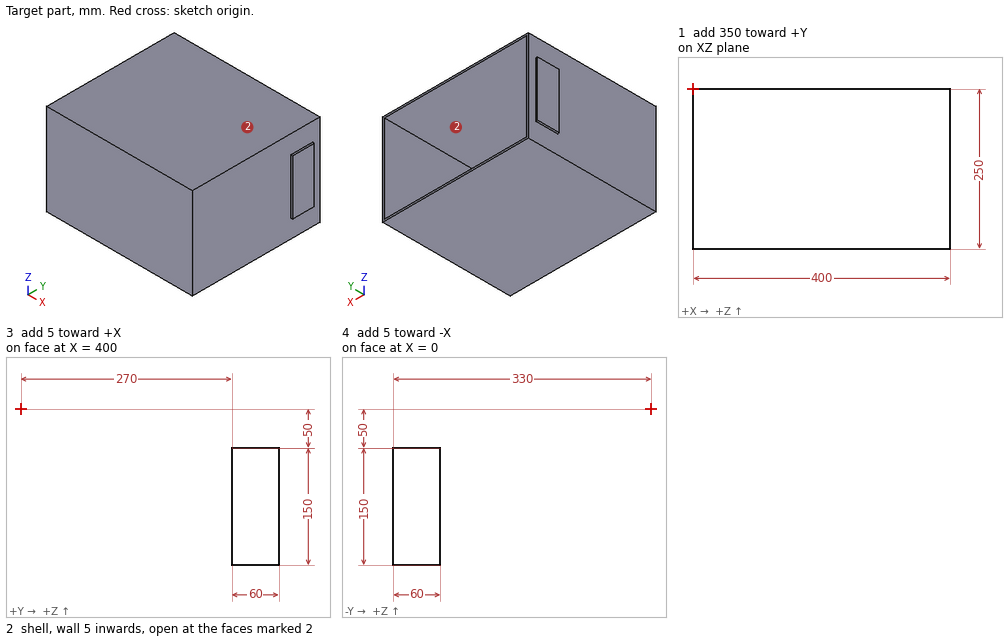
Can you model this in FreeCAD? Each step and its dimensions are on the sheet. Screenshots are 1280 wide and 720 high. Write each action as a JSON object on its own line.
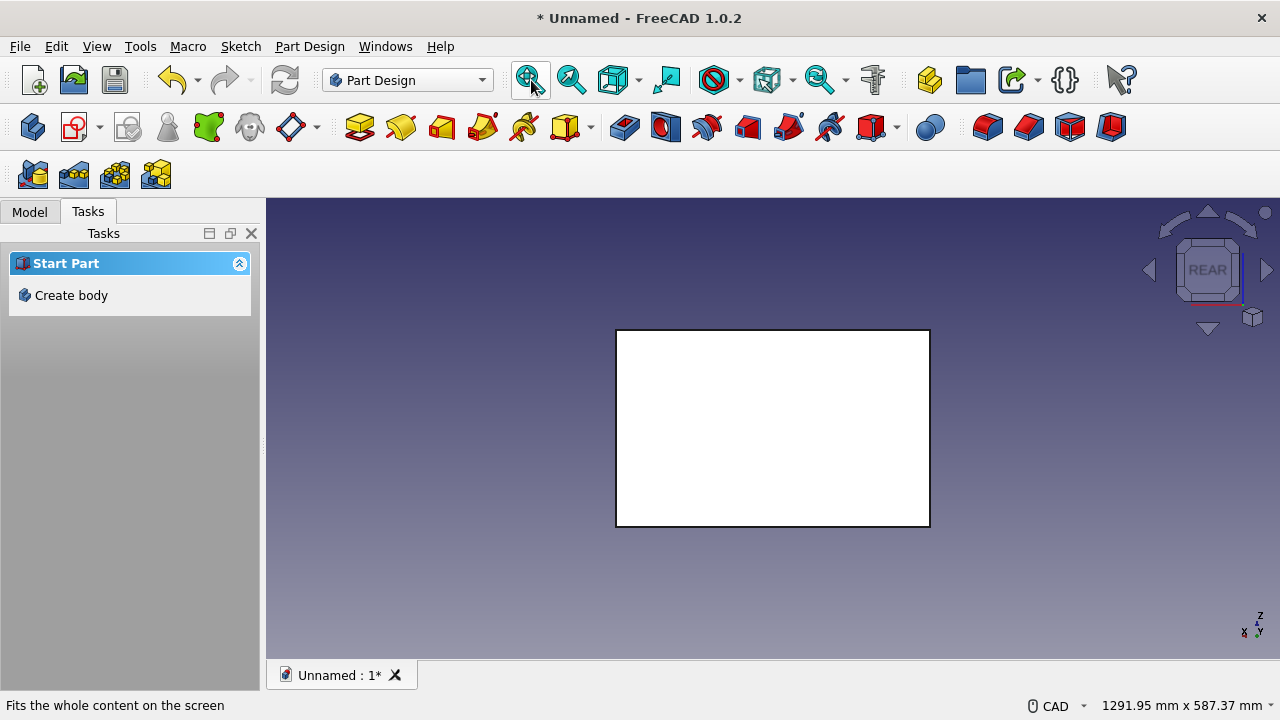
{"action": "key", "text": "v f"}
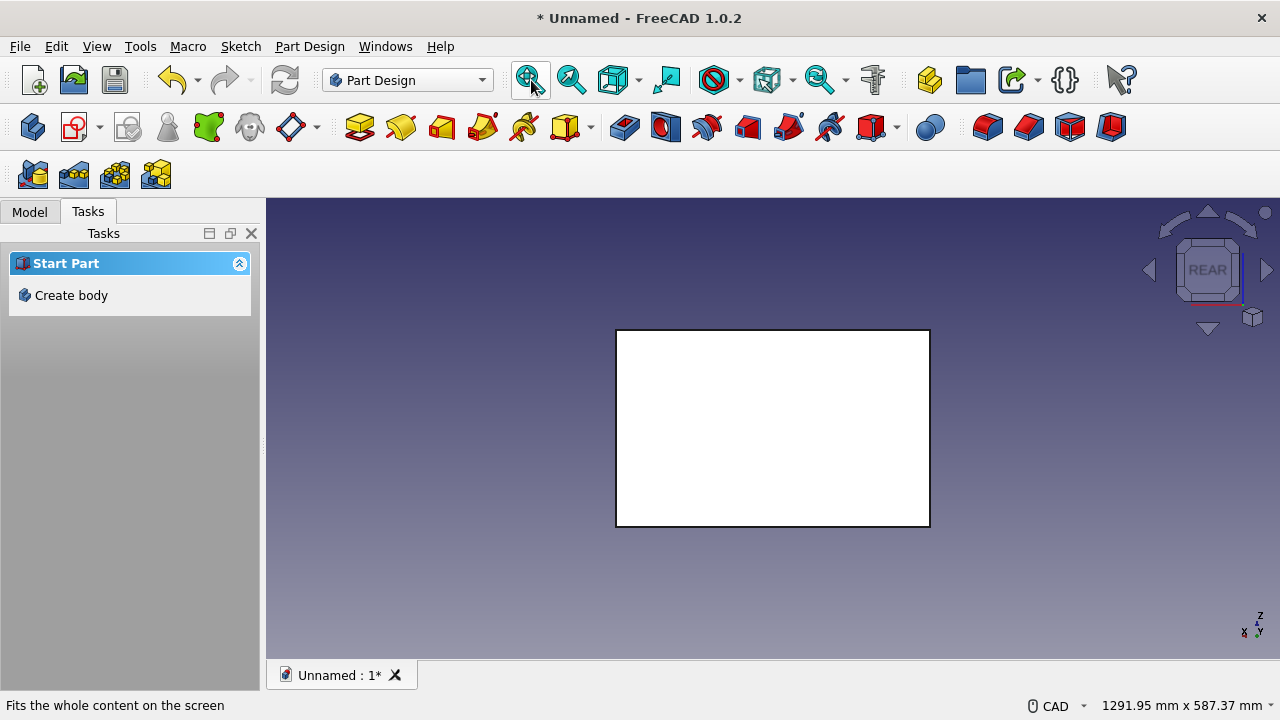
{"action": "left_click", "coordinate": [728, 428]}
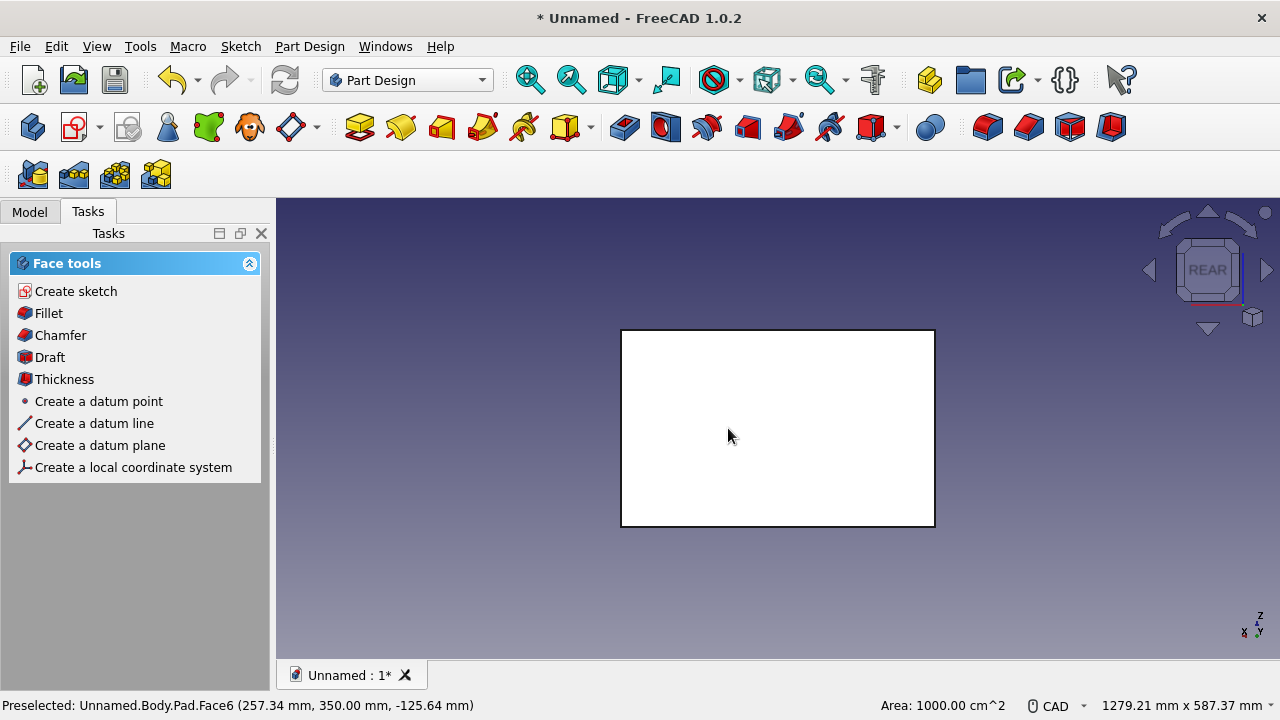
{"action": "left_click", "coordinate": [1111, 128]}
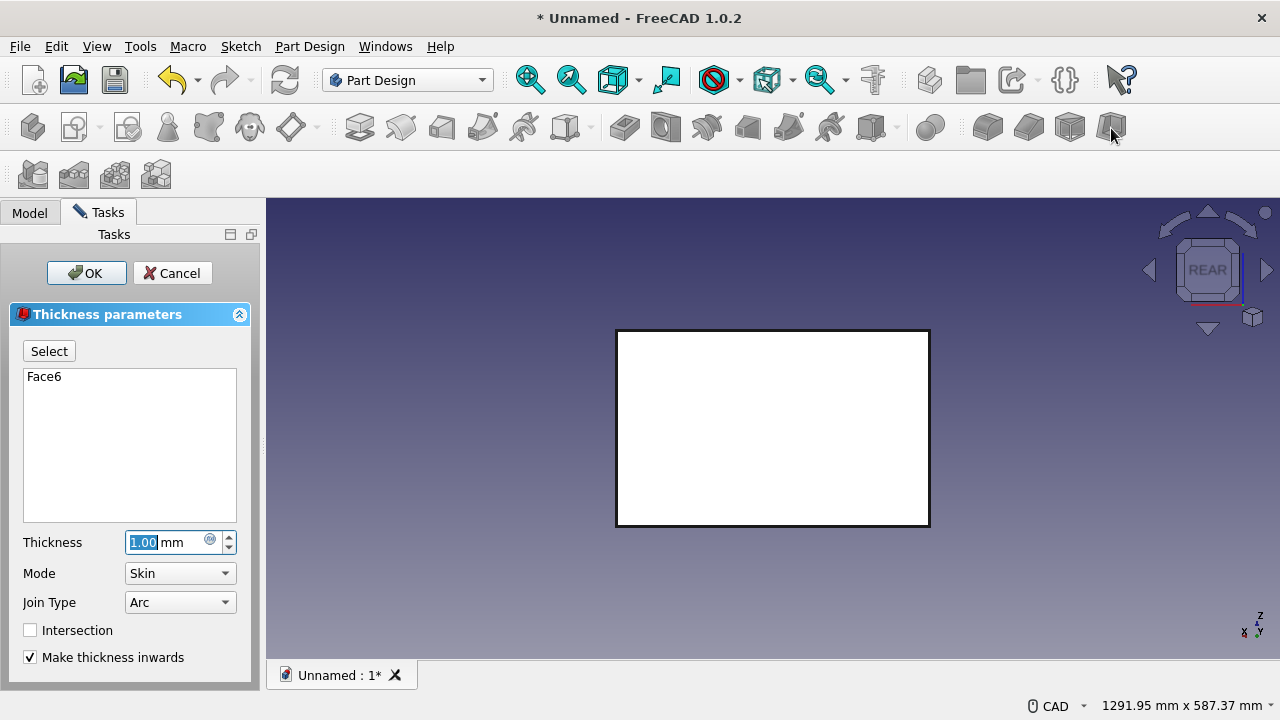
{"action": "type", "text": "5"}
{"action": "key", "text": "Tab"}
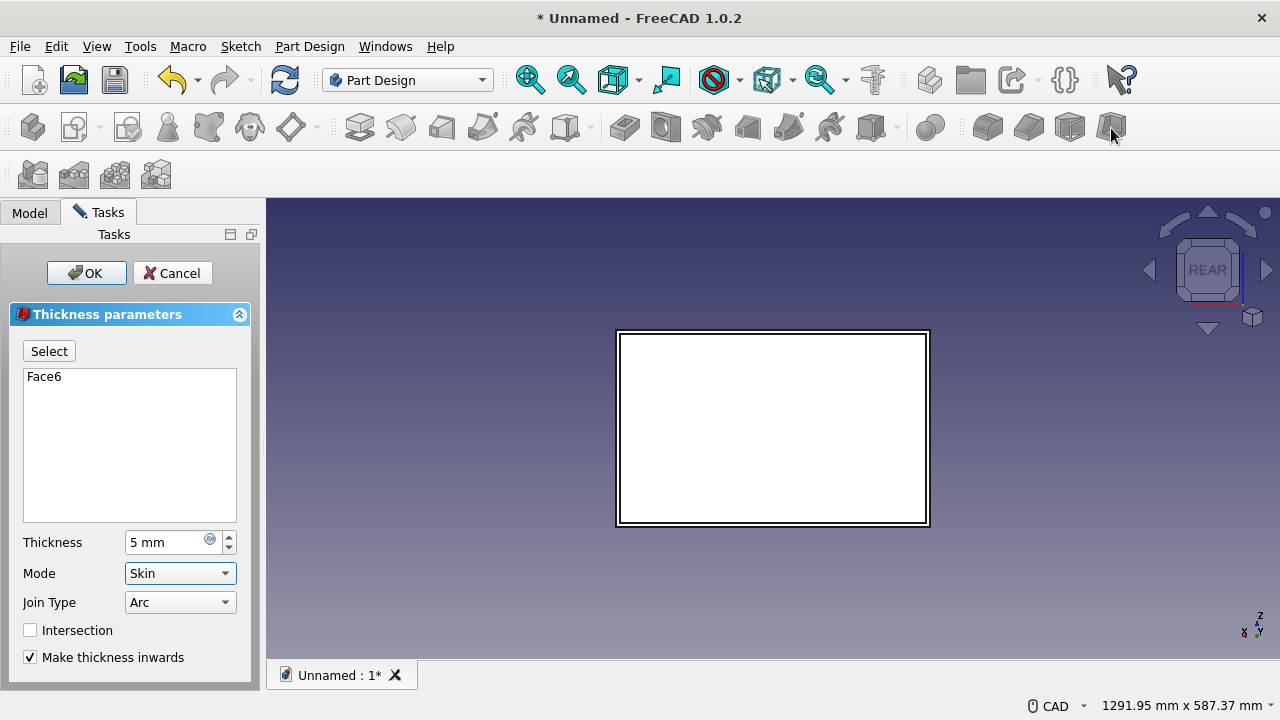
{"action": "left_click", "coordinate": [181, 602]}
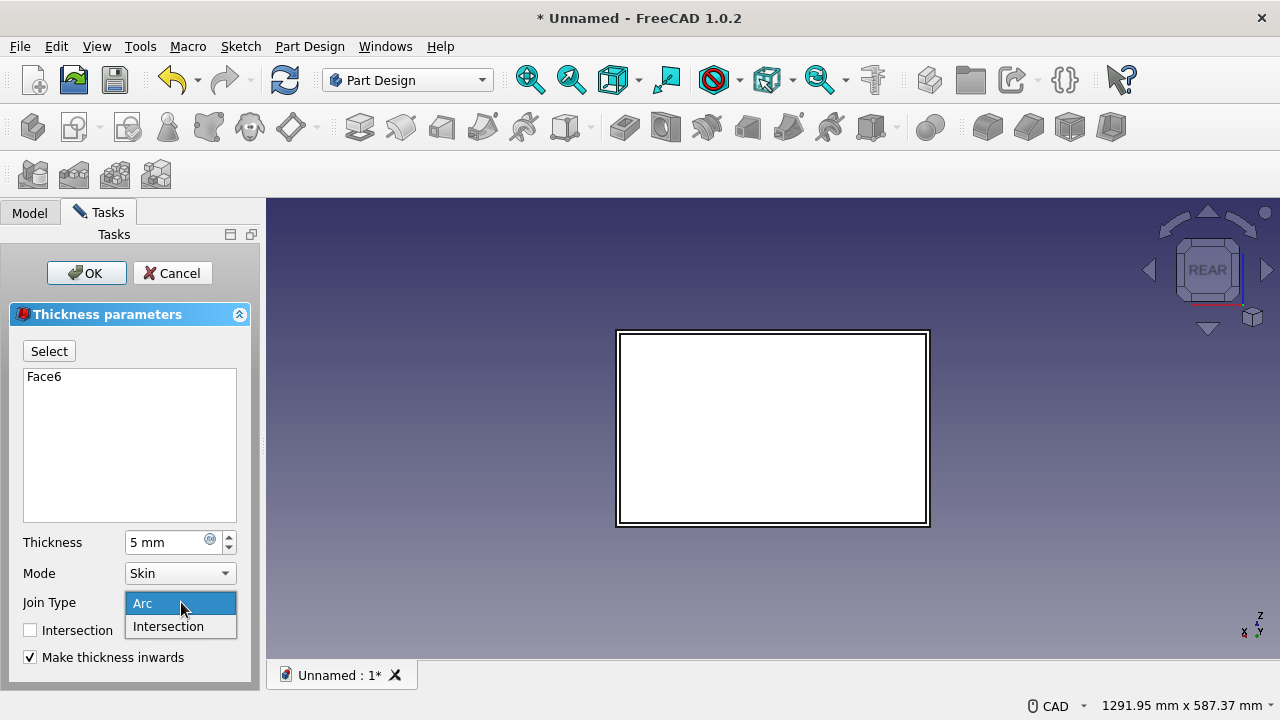
{"action": "left_click", "coordinate": [179, 626]}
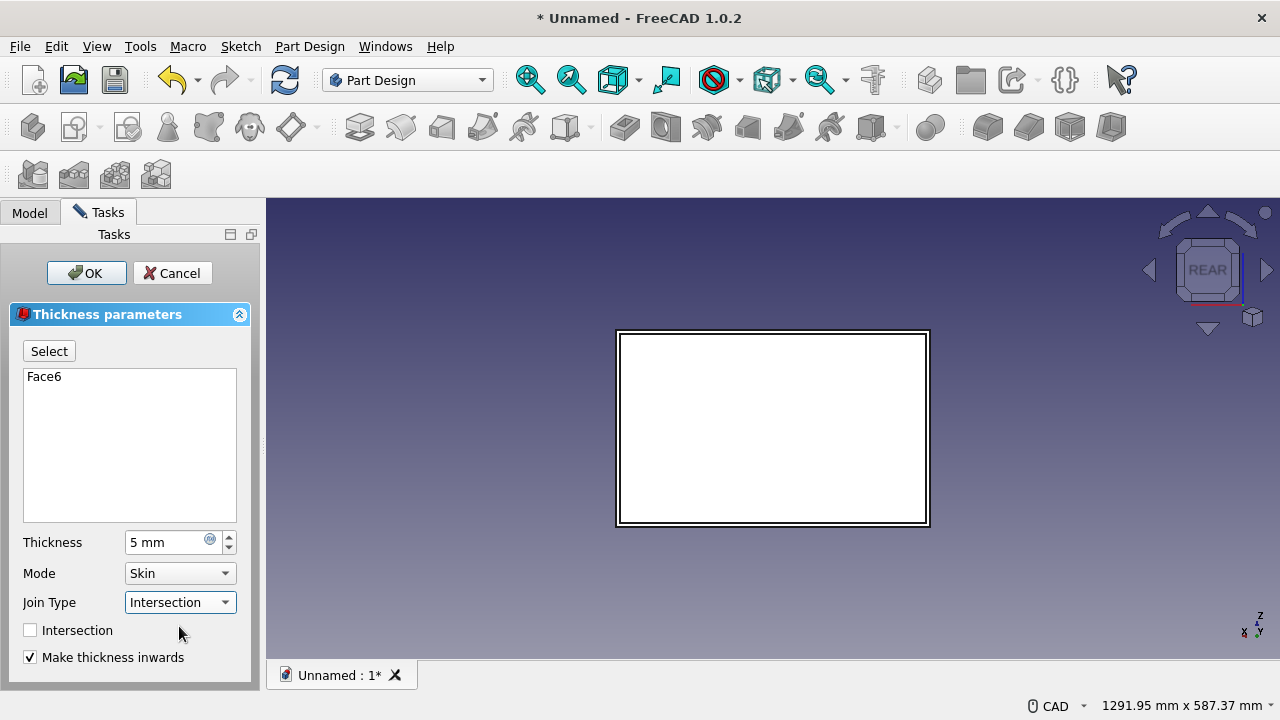
{"action": "left_click", "coordinate": [87, 273]}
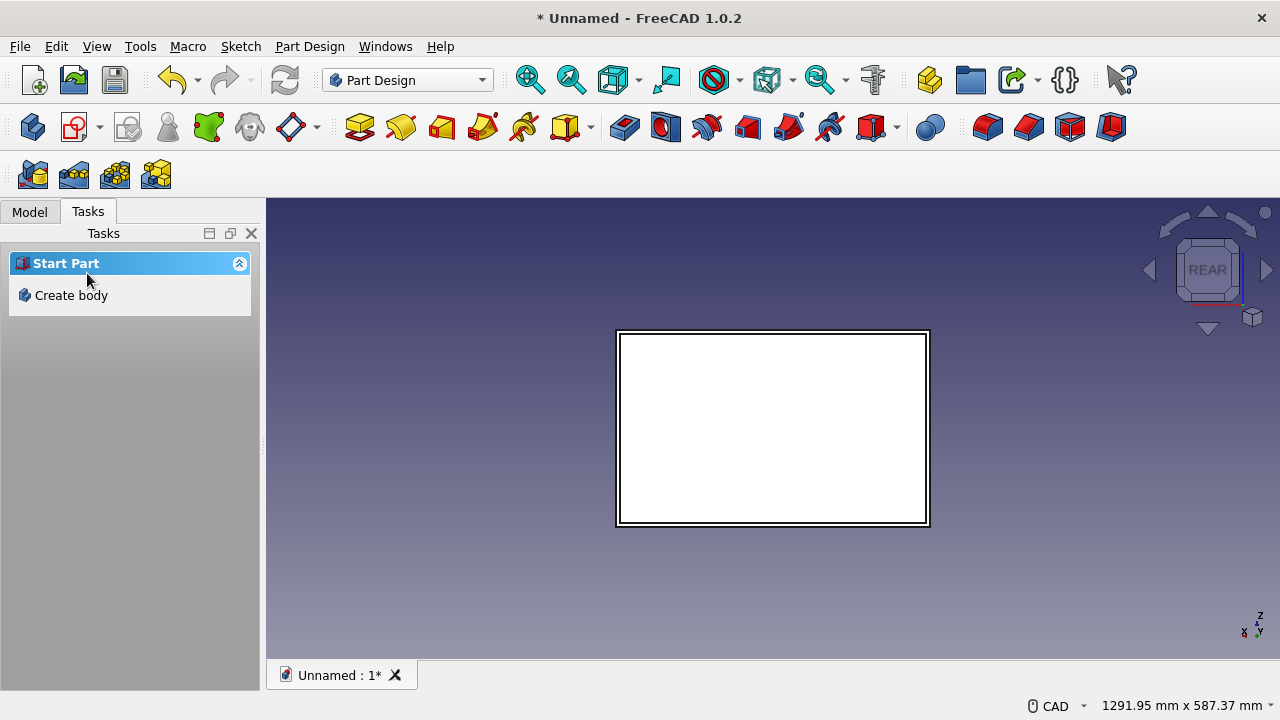
{"action": "key", "text": "v f"}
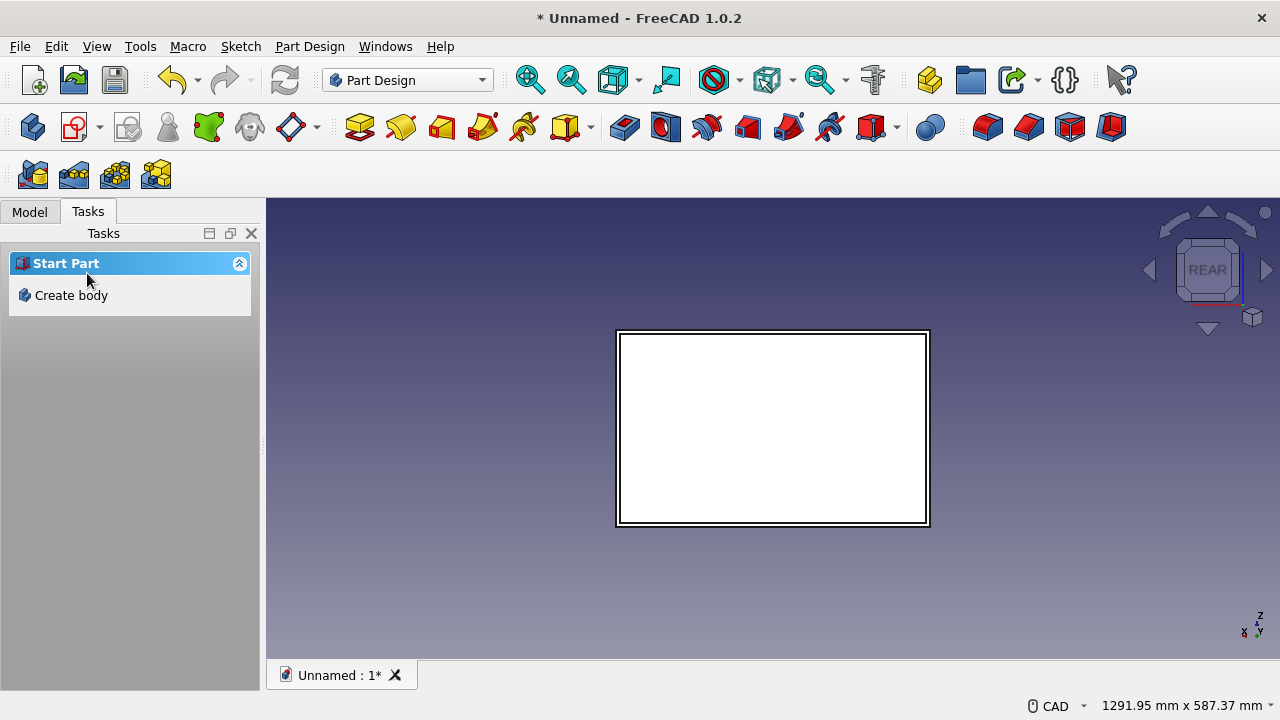
{"action": "key", "text": "0"}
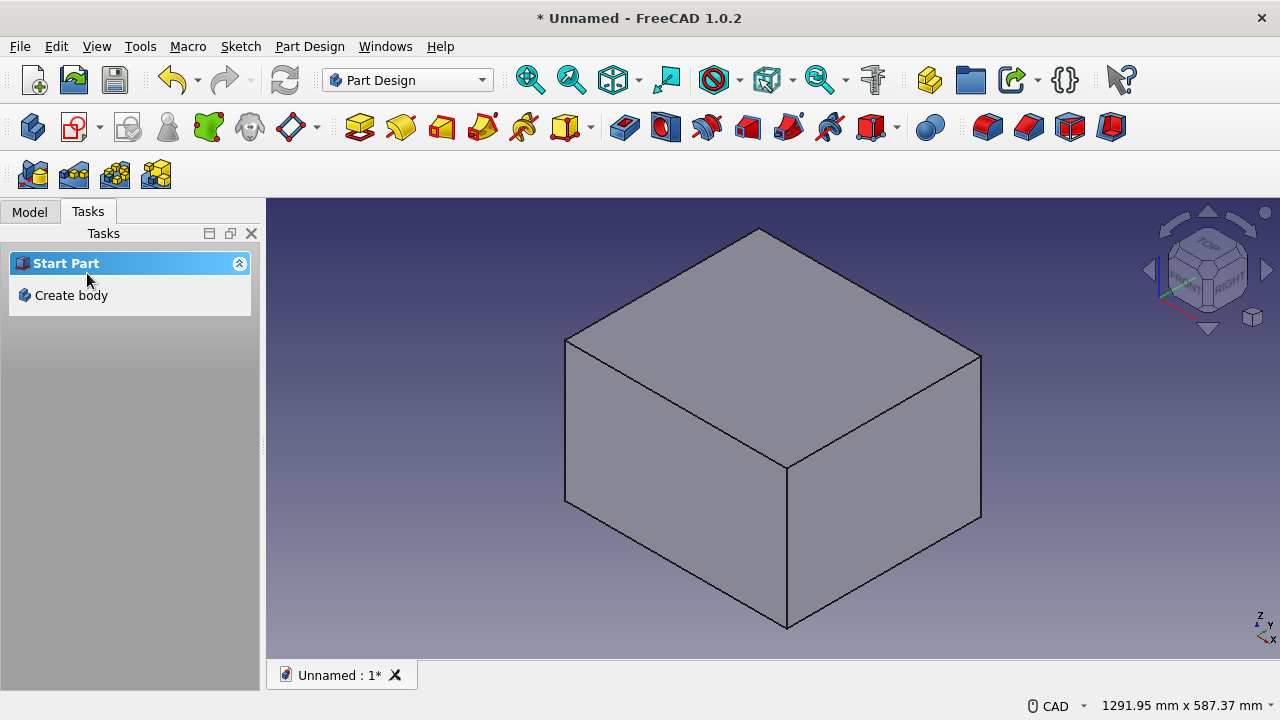
{"action": "left_click", "coordinate": [856, 508]}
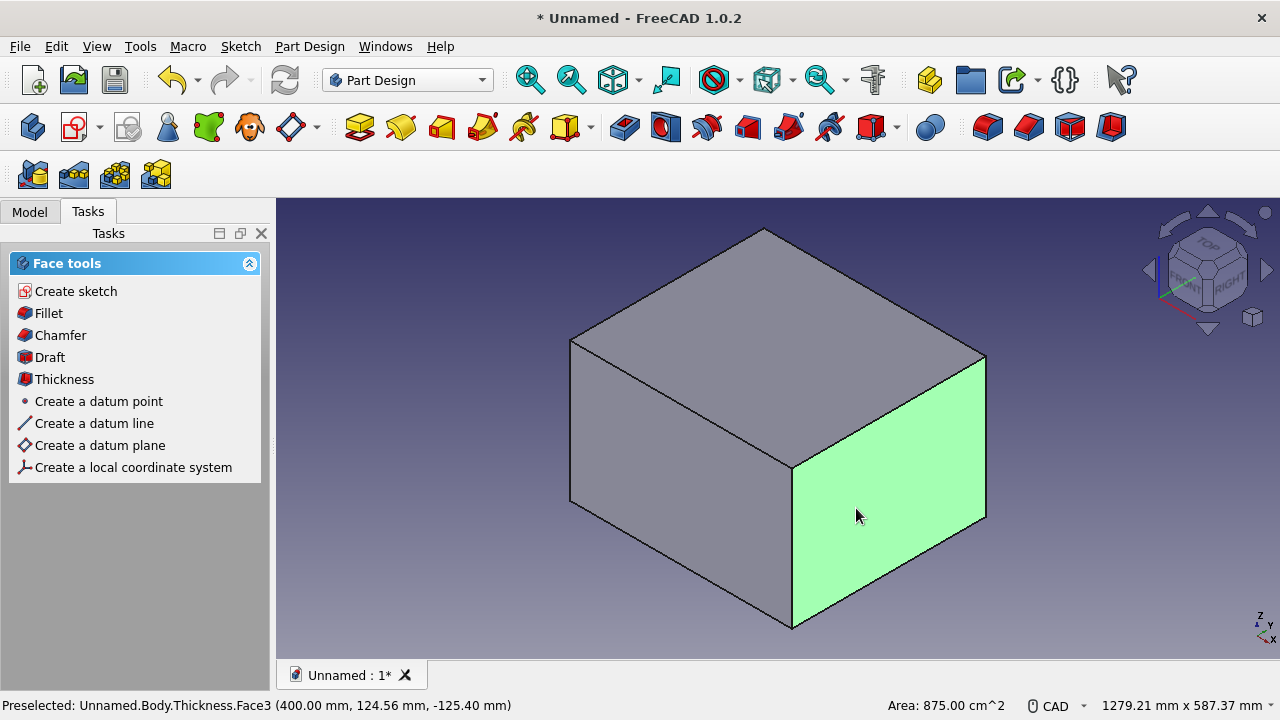
{"action": "left_click", "coordinate": [74, 128]}